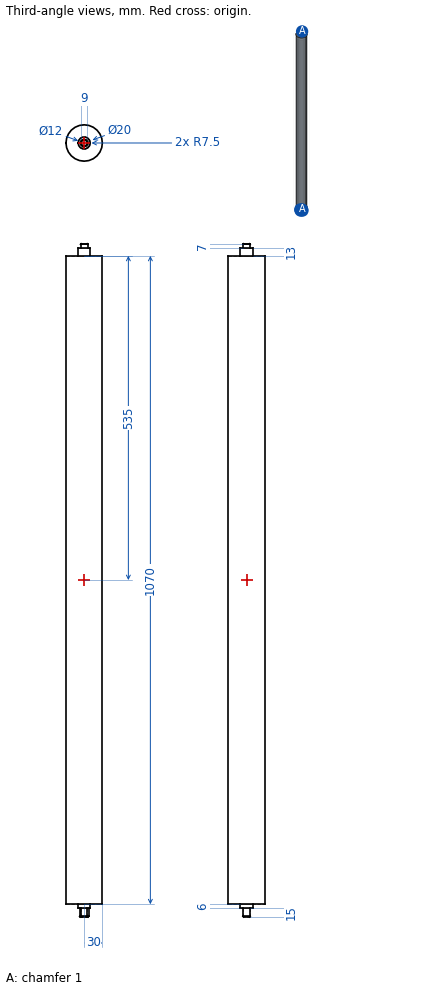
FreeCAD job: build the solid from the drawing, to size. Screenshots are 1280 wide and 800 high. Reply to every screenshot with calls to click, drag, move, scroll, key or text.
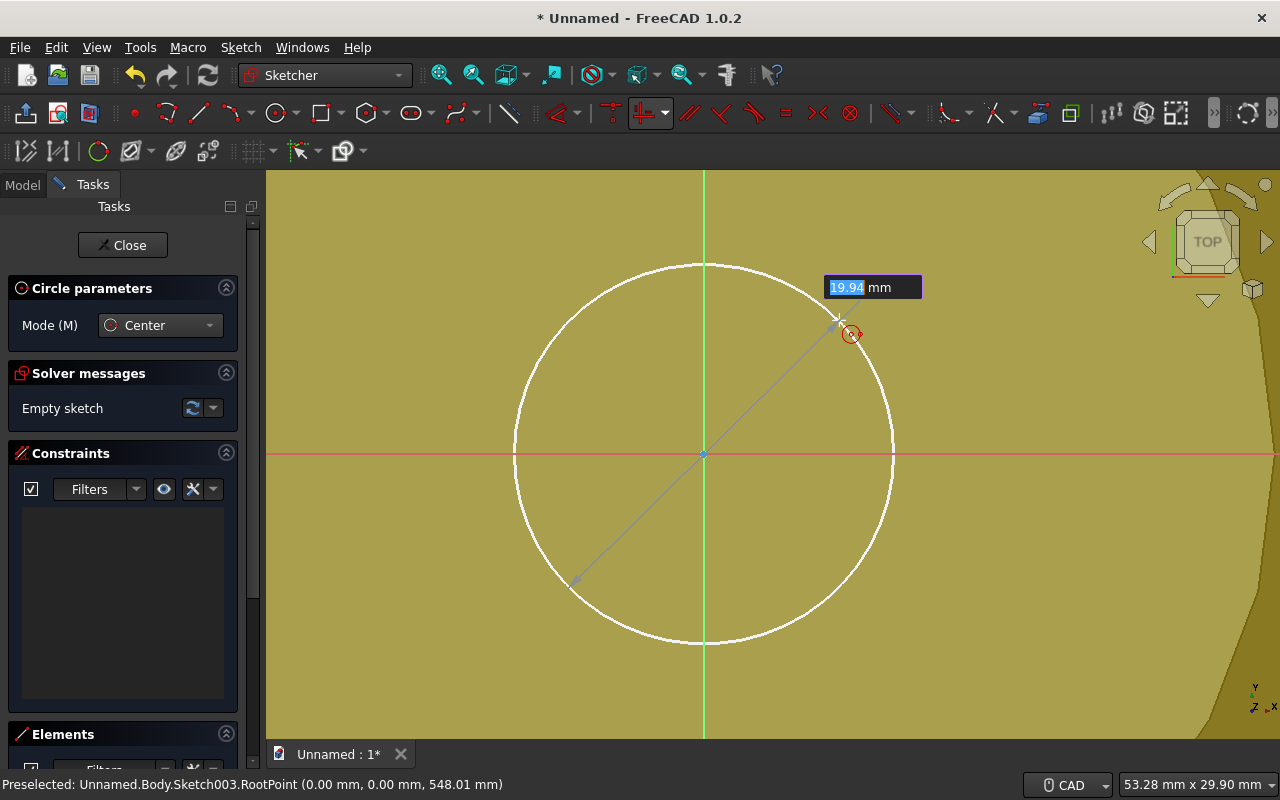
text(20)
key(Return)
key(Escape)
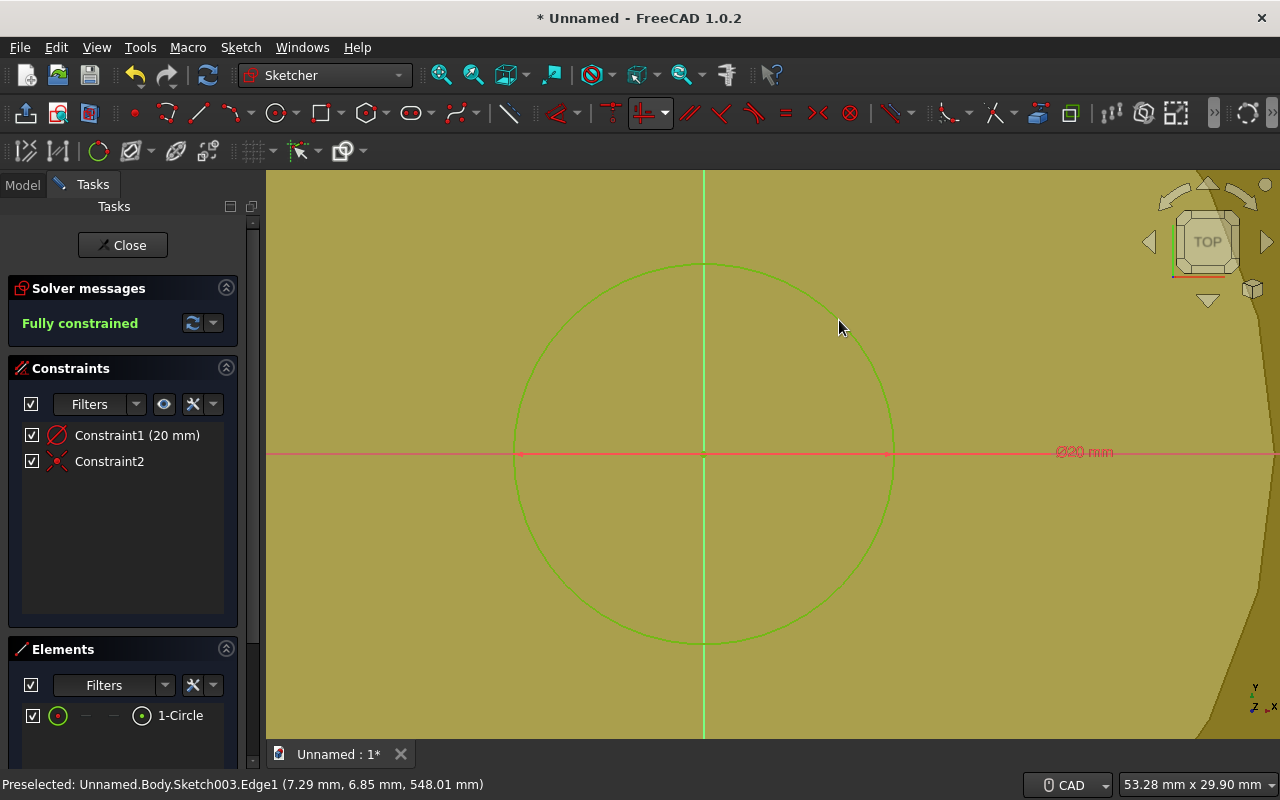
click(123, 245)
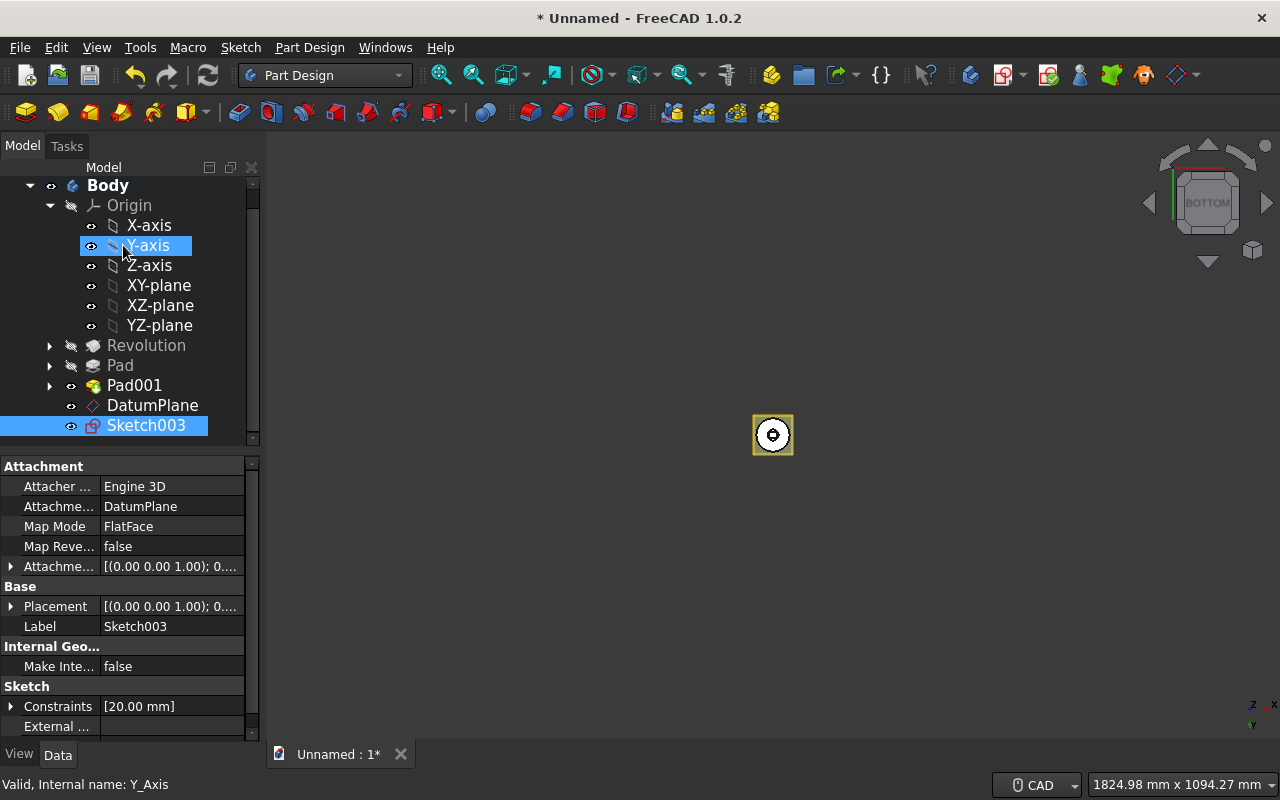
click(26, 112)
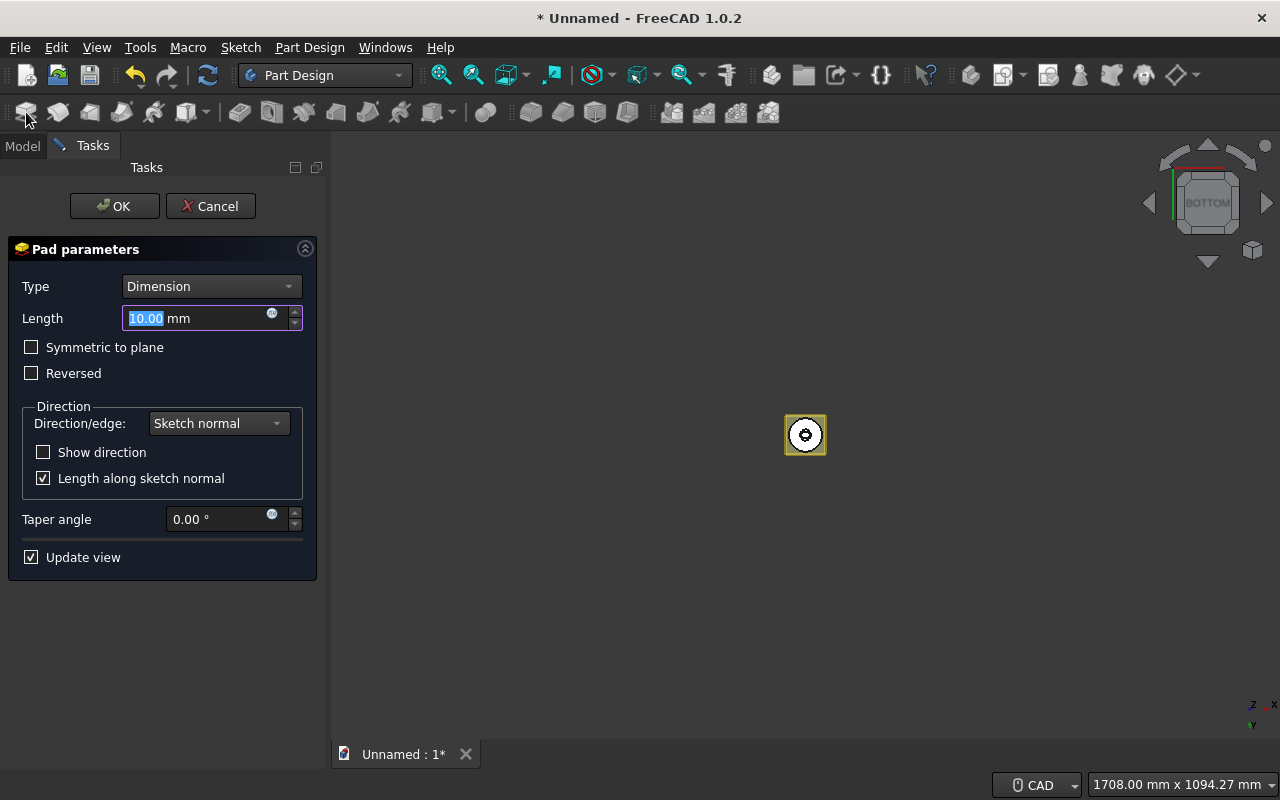
text(13)
key(Tab)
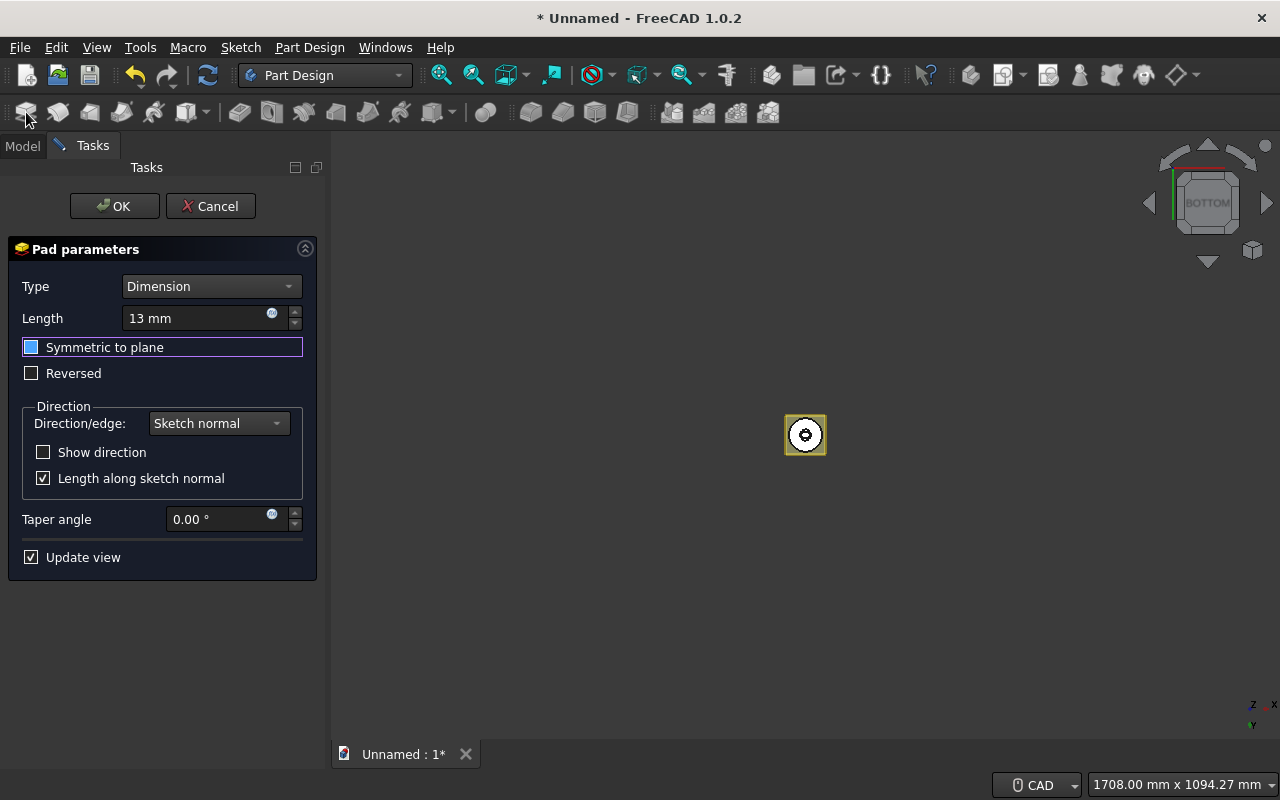
click(30, 373)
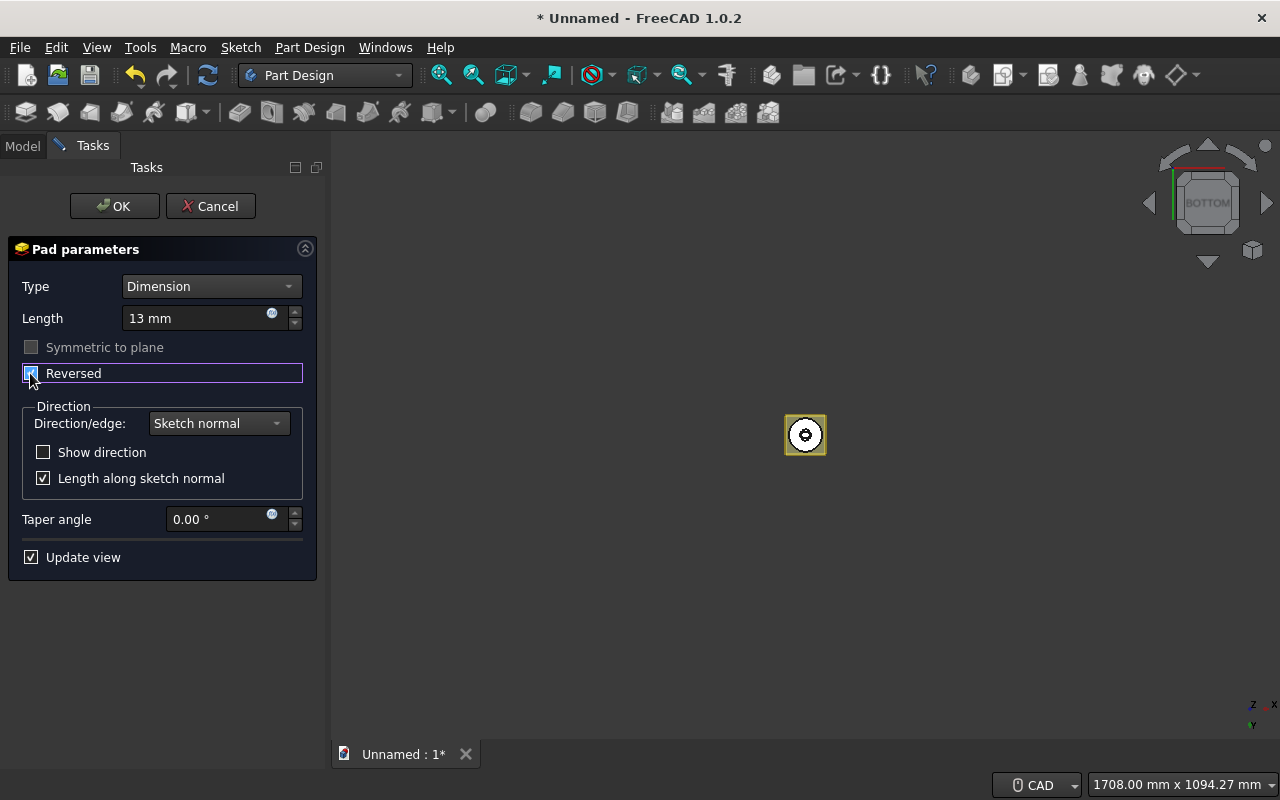
click(115, 206)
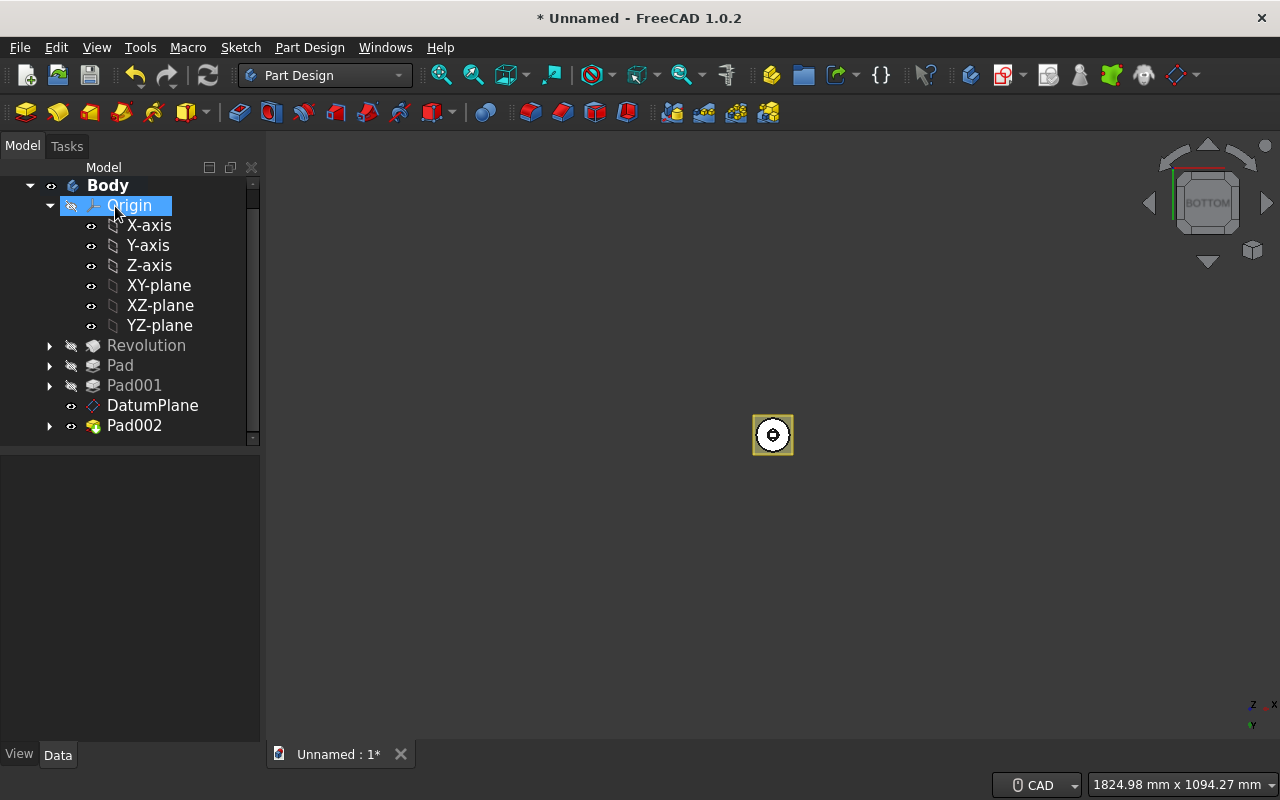
click(116, 406)
key(space)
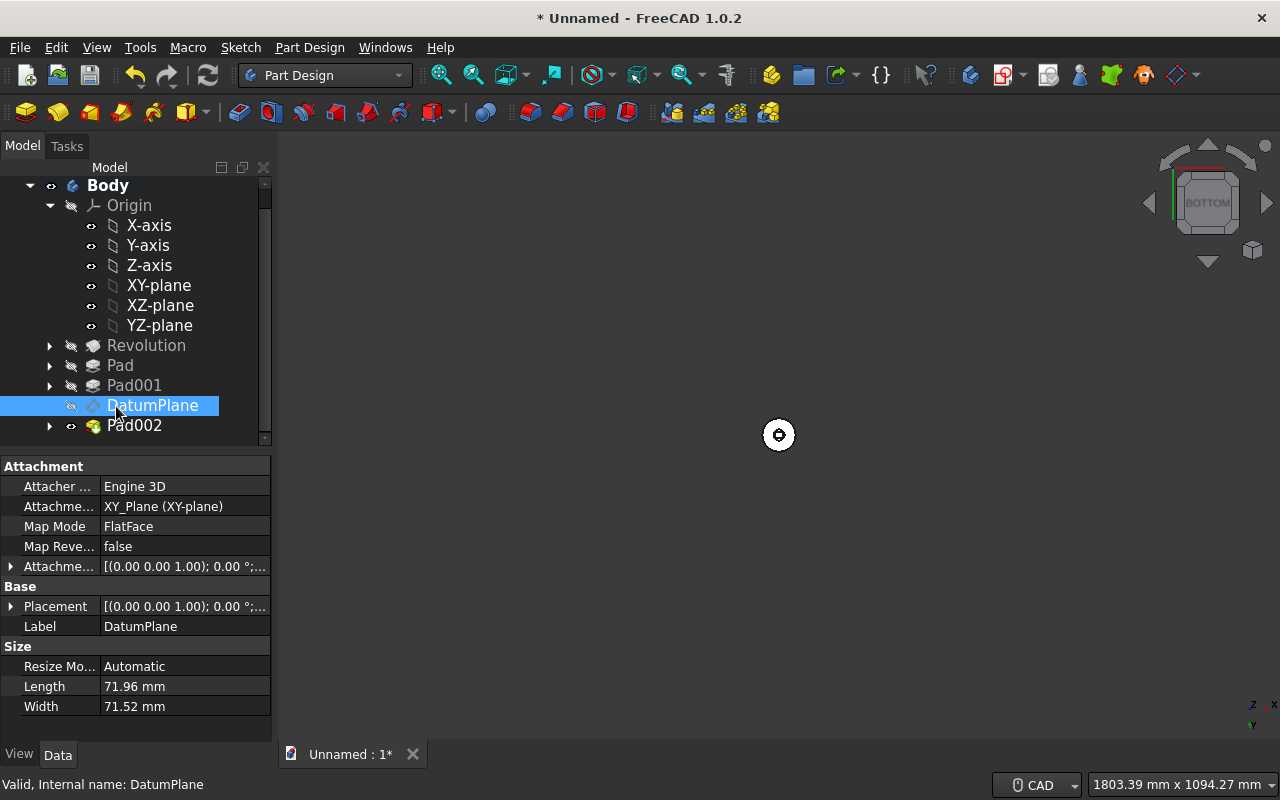
click(442, 76)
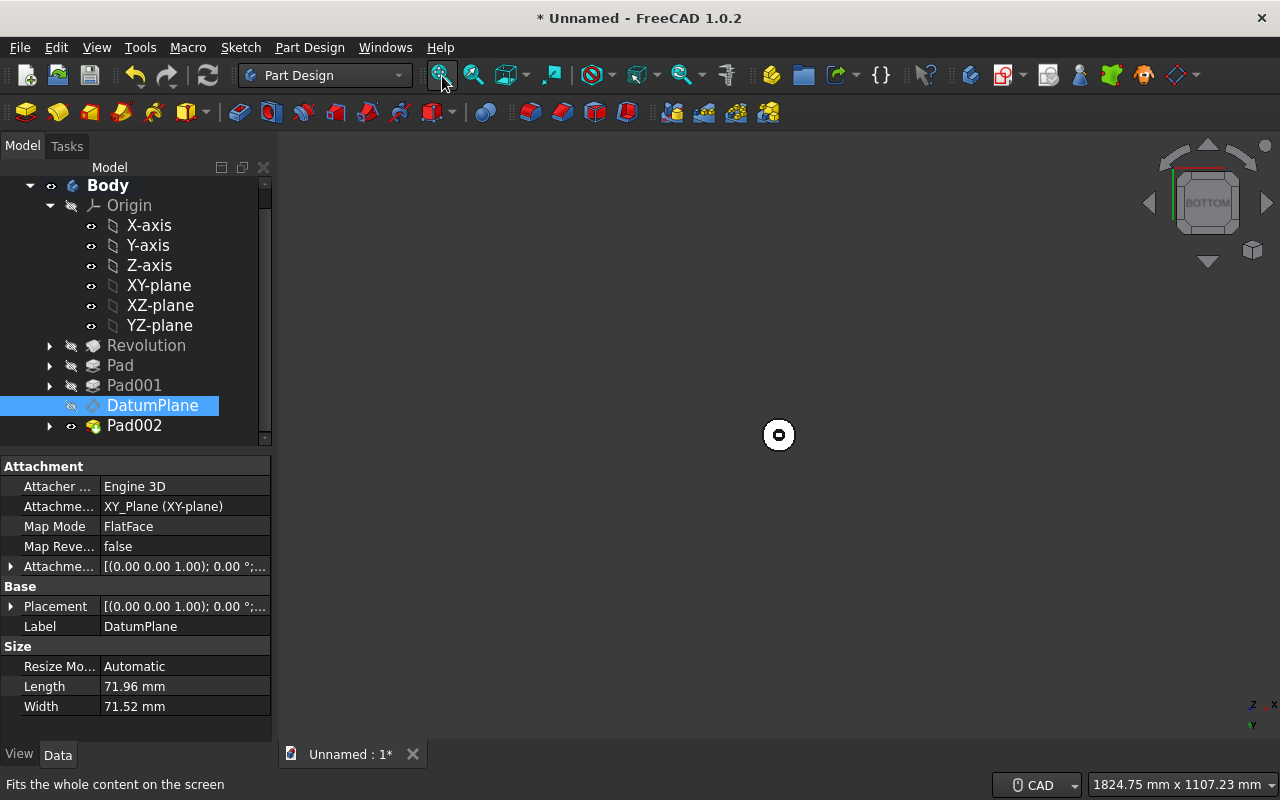
key(0)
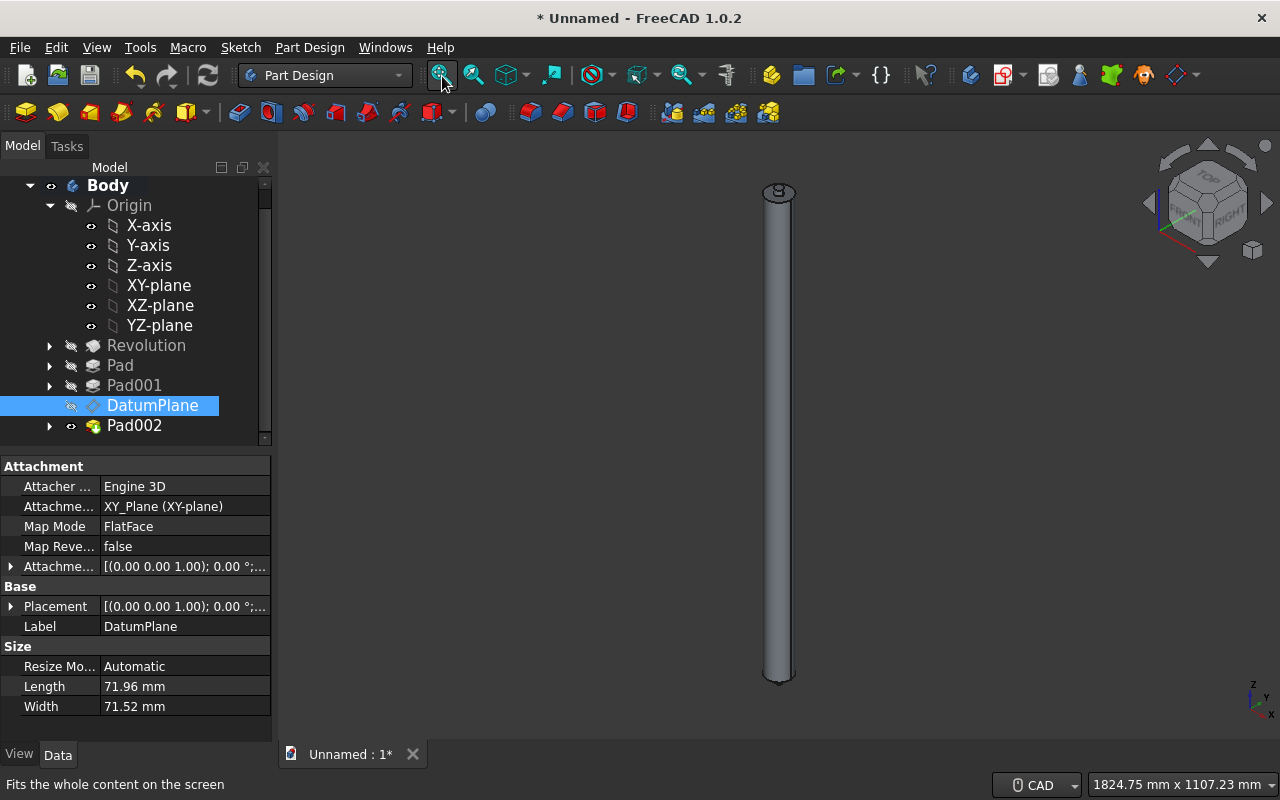
scroll(779, 187, up, 4)